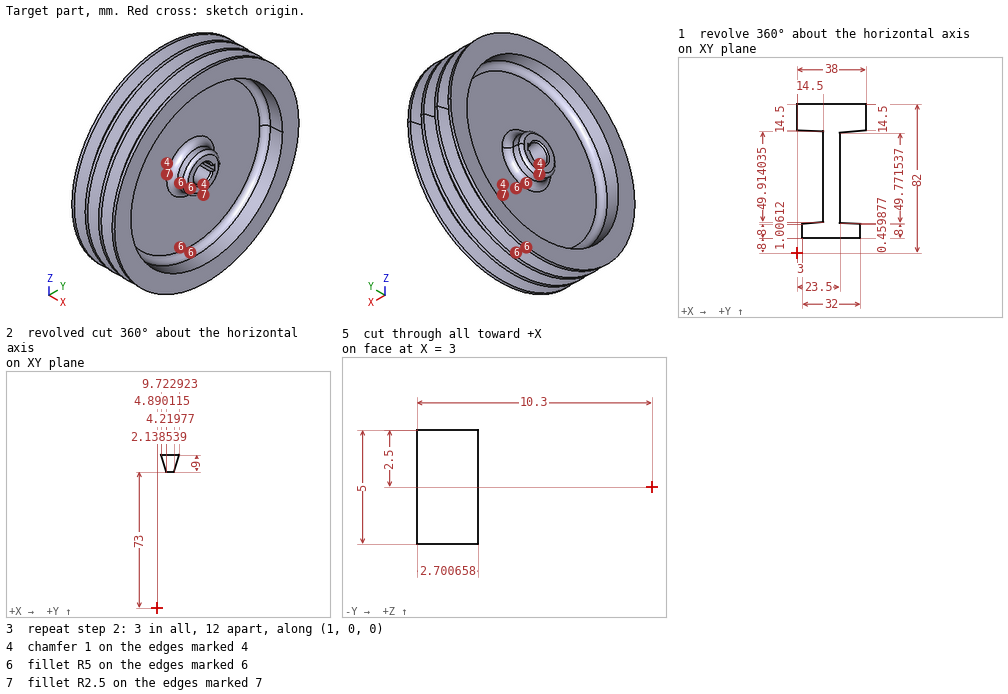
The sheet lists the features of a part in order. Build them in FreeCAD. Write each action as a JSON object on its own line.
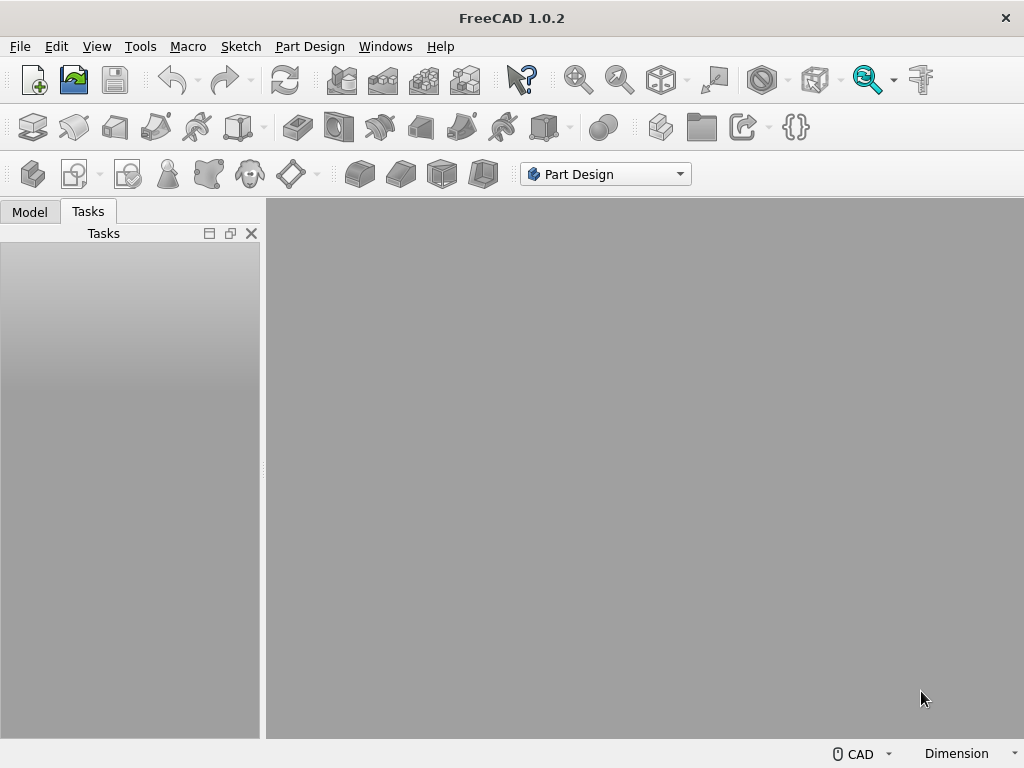
{"action": "left_click", "coordinate": [33, 80]}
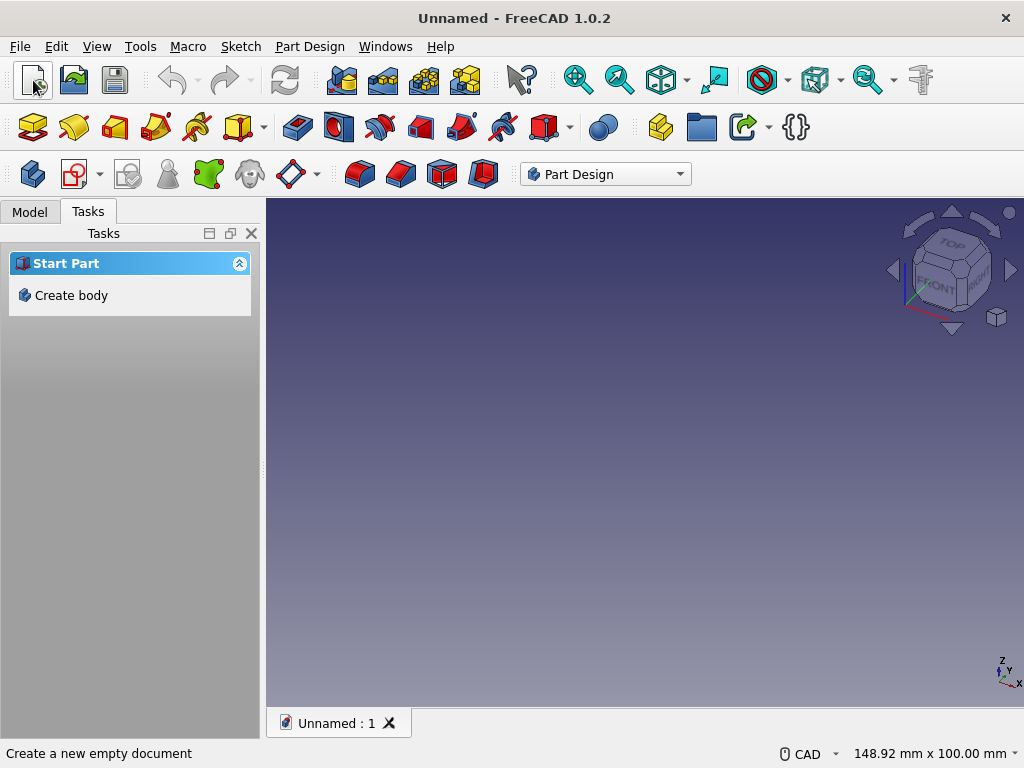
{"action": "left_click", "coordinate": [74, 174]}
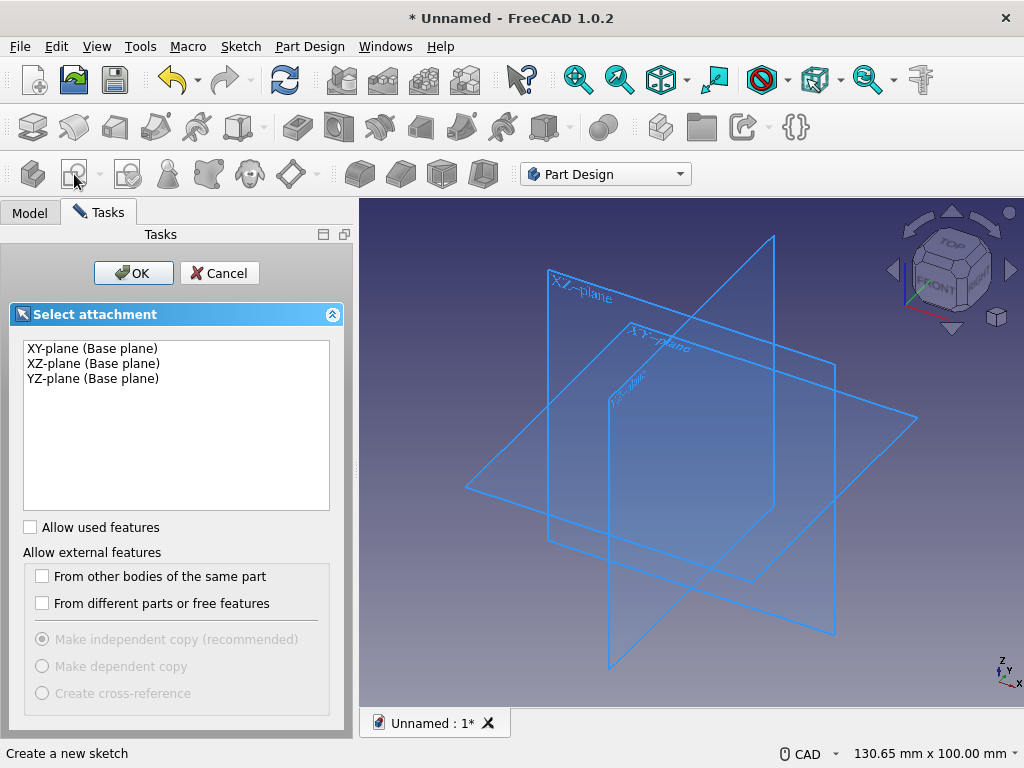
{"action": "left_click", "coordinate": [84, 348]}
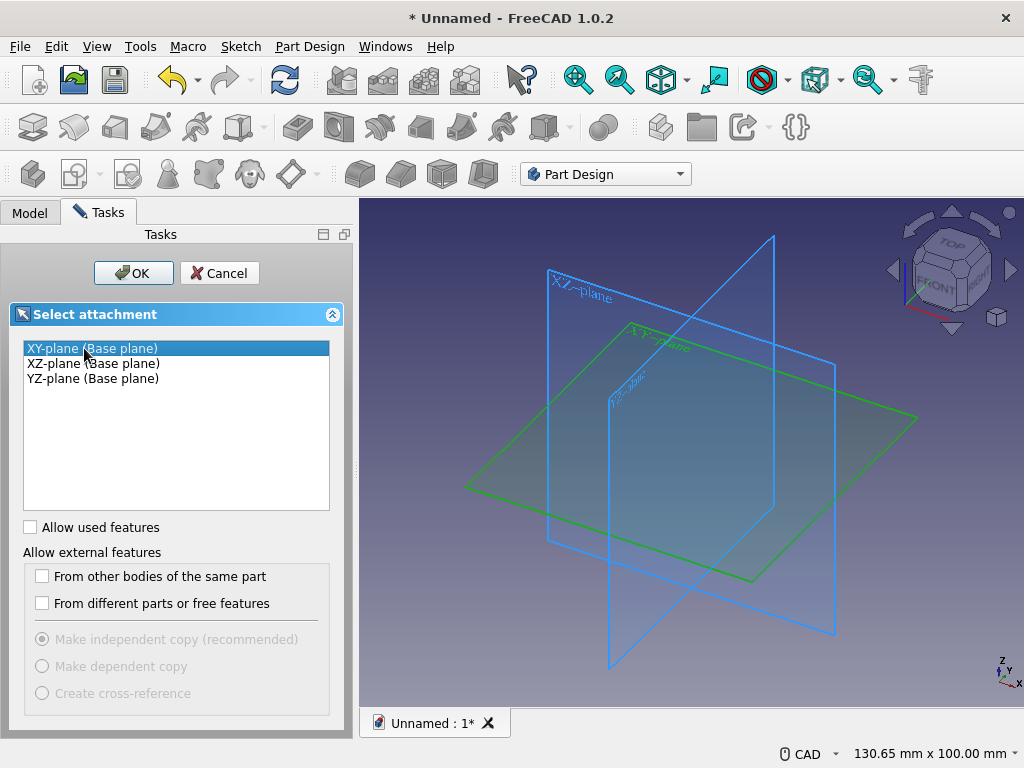
{"action": "left_click", "coordinate": [134, 273]}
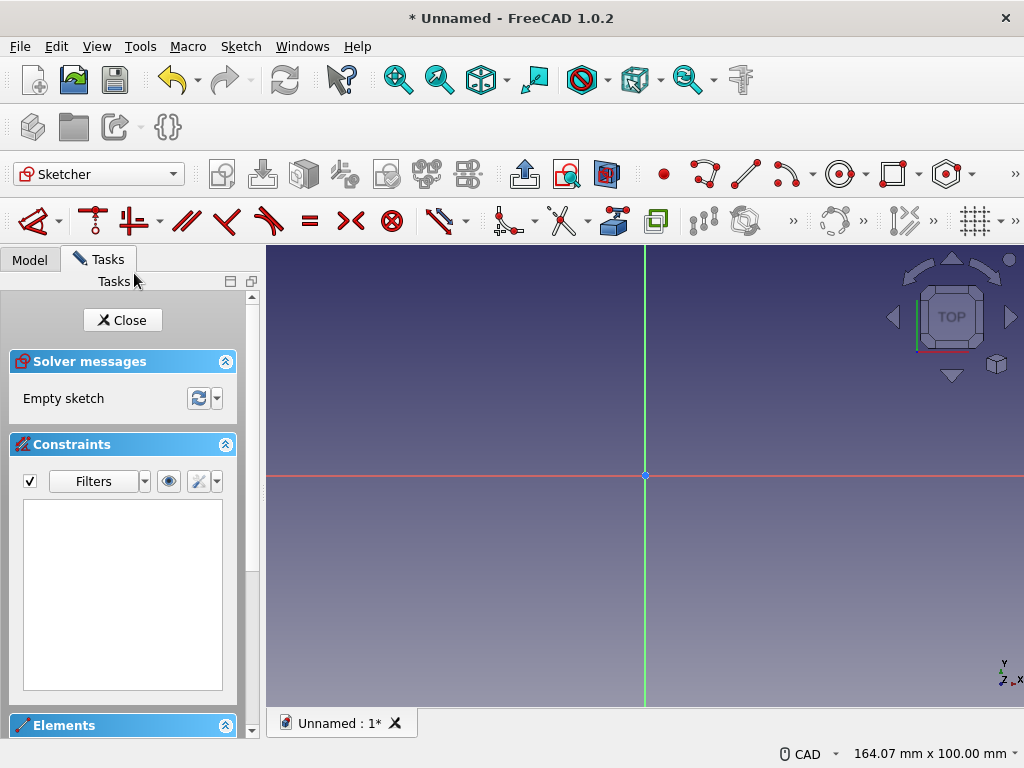
{"action": "scroll", "coordinate": [386, 679], "scroll_direction": "down", "scroll_amount": 3}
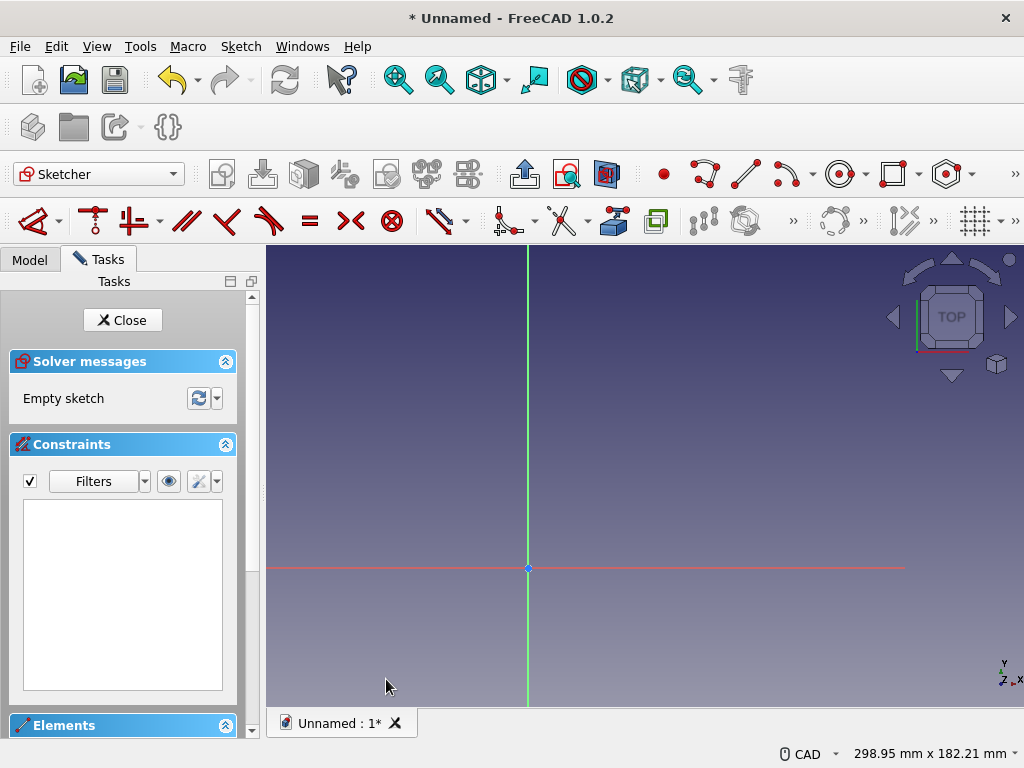
{"action": "scroll", "coordinate": [576, 440], "scroll_direction": "up", "scroll_amount": 2}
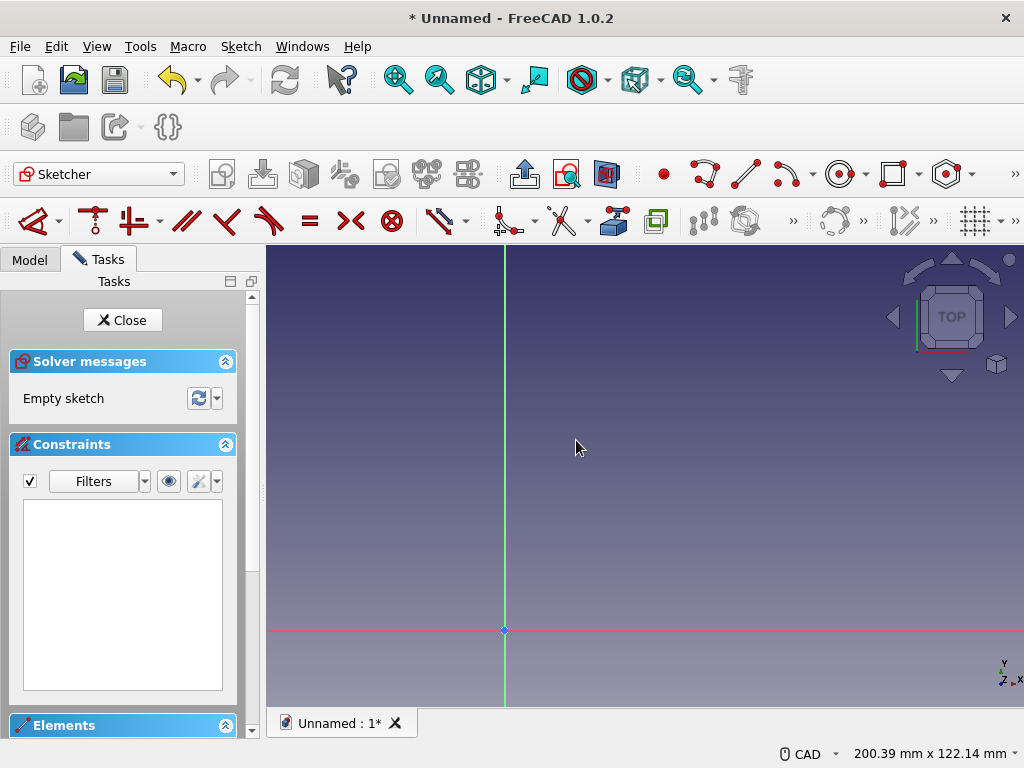
{"action": "left_click", "coordinate": [705, 174]}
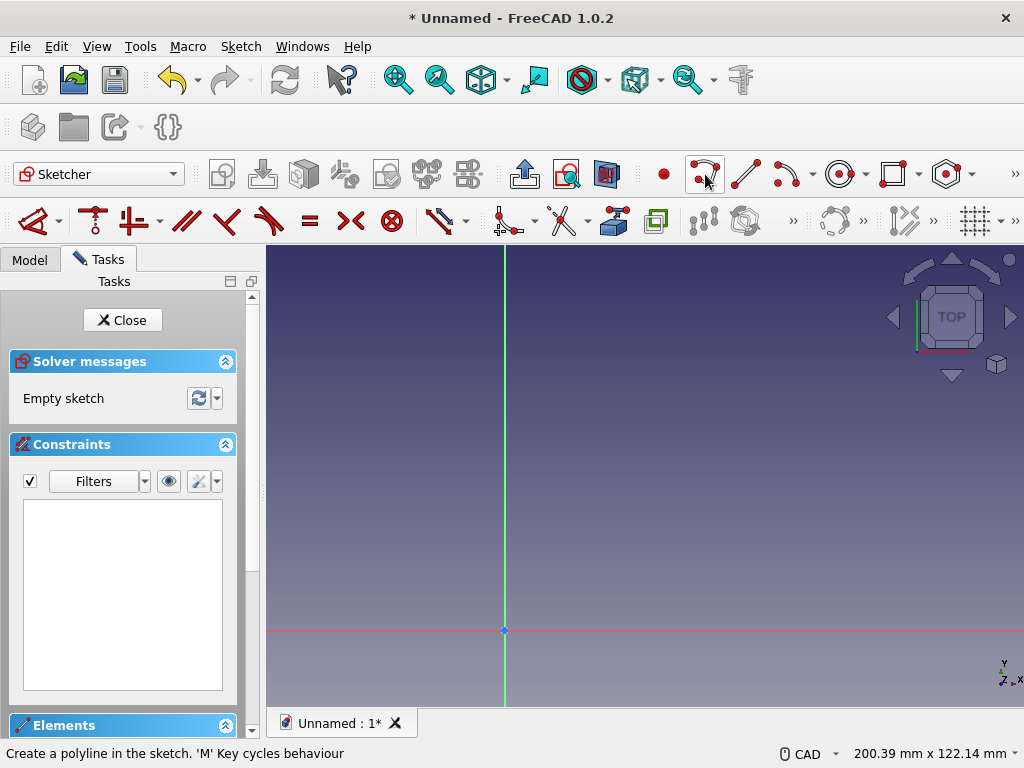
{"action": "scroll", "coordinate": [516, 601], "scroll_direction": "up", "scroll_amount": 2}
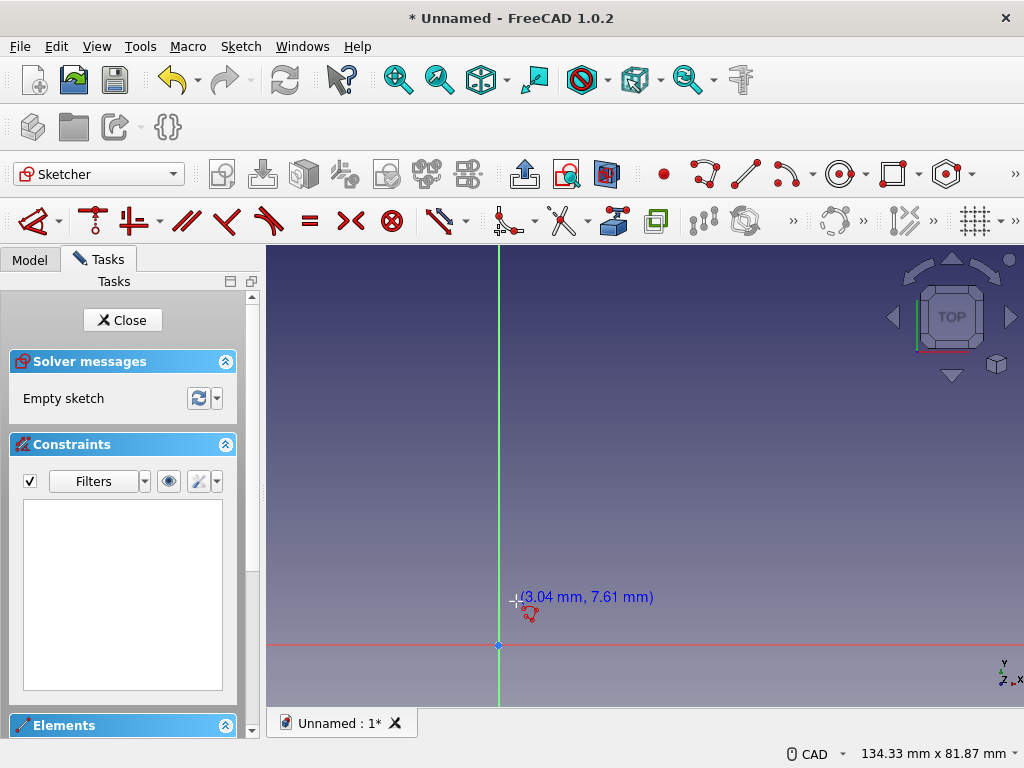
{"action": "left_click", "coordinate": [516, 600]}
{"action": "left_click", "coordinate": [696, 600]}
{"action": "left_click", "coordinate": [696, 555]}
{"action": "left_click", "coordinate": [631, 551]}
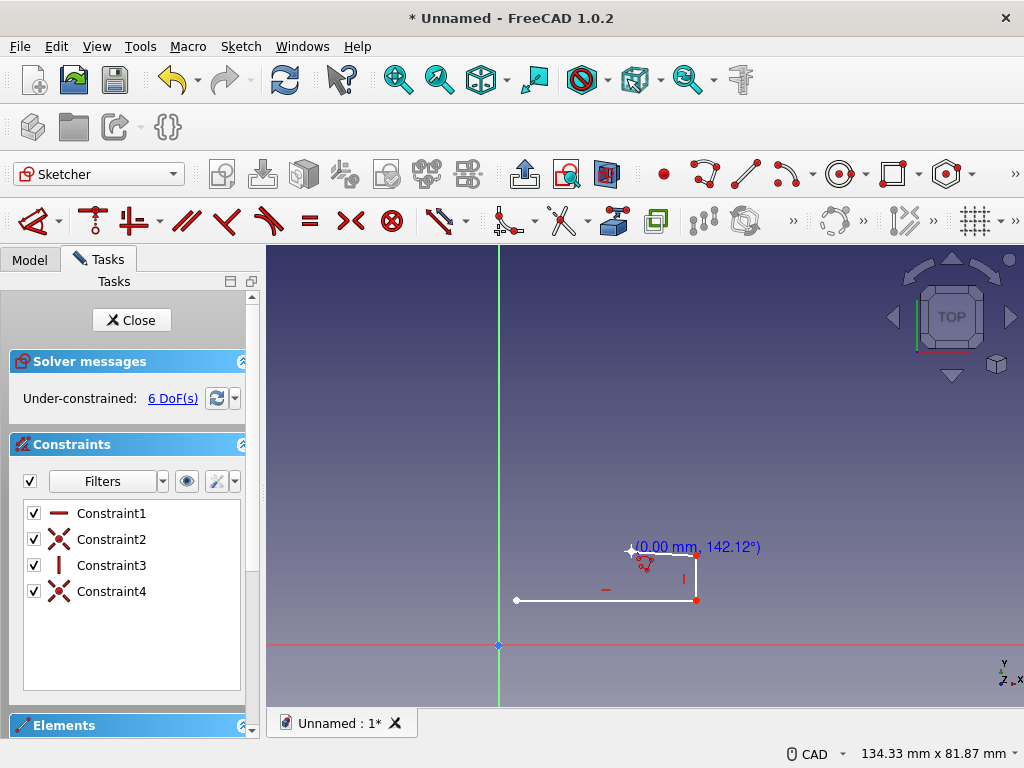
{"action": "scroll", "coordinate": [517, 603], "scroll_direction": "down", "scroll_amount": 2}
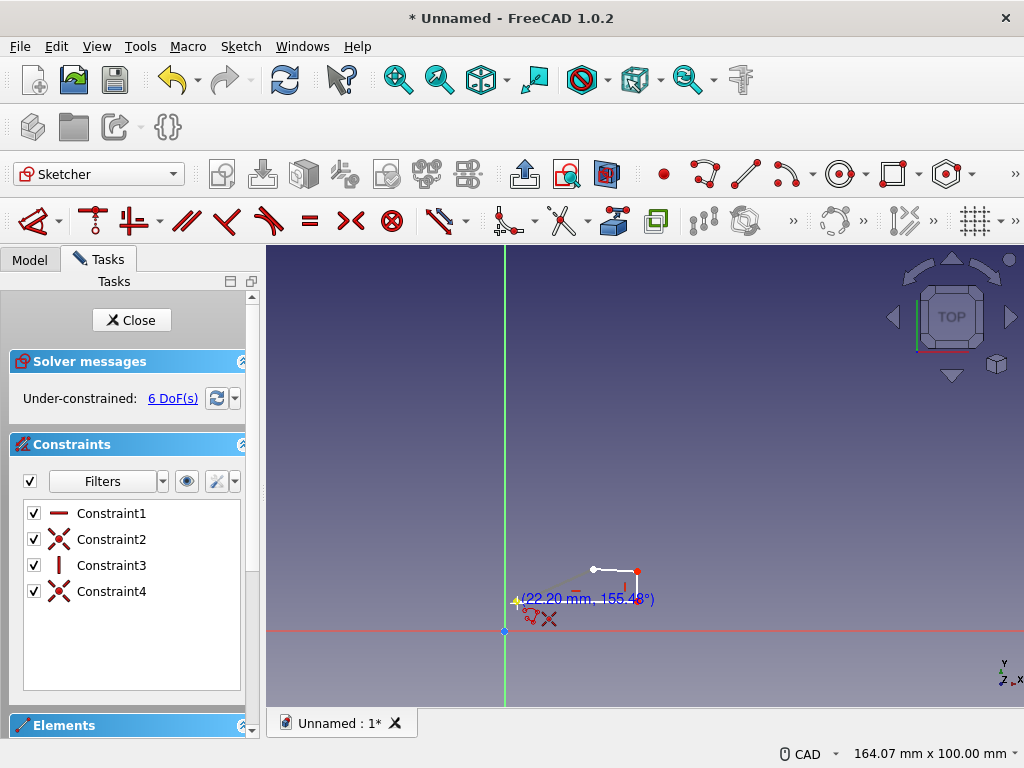
{"action": "left_click", "coordinate": [594, 381]}
{"action": "left_click", "coordinate": [649, 376]}
{"action": "left_click", "coordinate": [649, 321]}
{"action": "left_click", "coordinate": [505, 321]}
{"action": "left_click", "coordinate": [514, 376]}
{"action": "left_click", "coordinate": [560, 380]}
{"action": "left_click", "coordinate": [560, 567]}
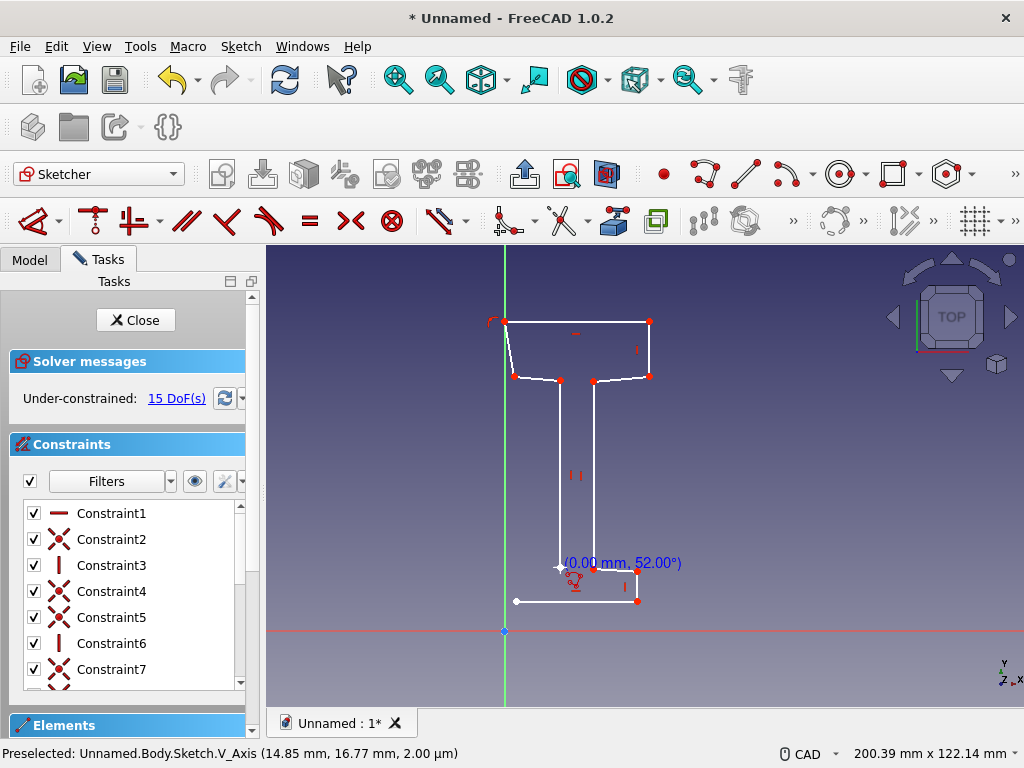
{"action": "scroll", "coordinate": [516, 571], "scroll_direction": "up", "scroll_amount": 2}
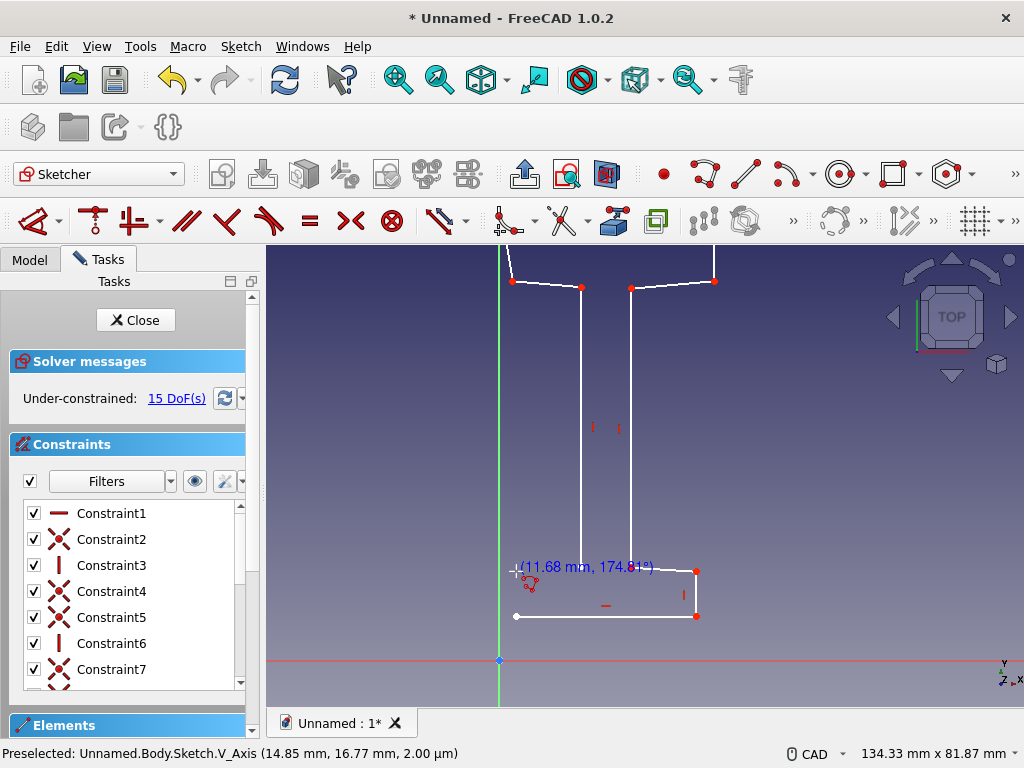
{"action": "left_click", "coordinate": [516, 571]}
{"action": "left_click", "coordinate": [516, 617]}
{"action": "key", "text": "Escape"}
{"action": "key", "text": "Escape"}